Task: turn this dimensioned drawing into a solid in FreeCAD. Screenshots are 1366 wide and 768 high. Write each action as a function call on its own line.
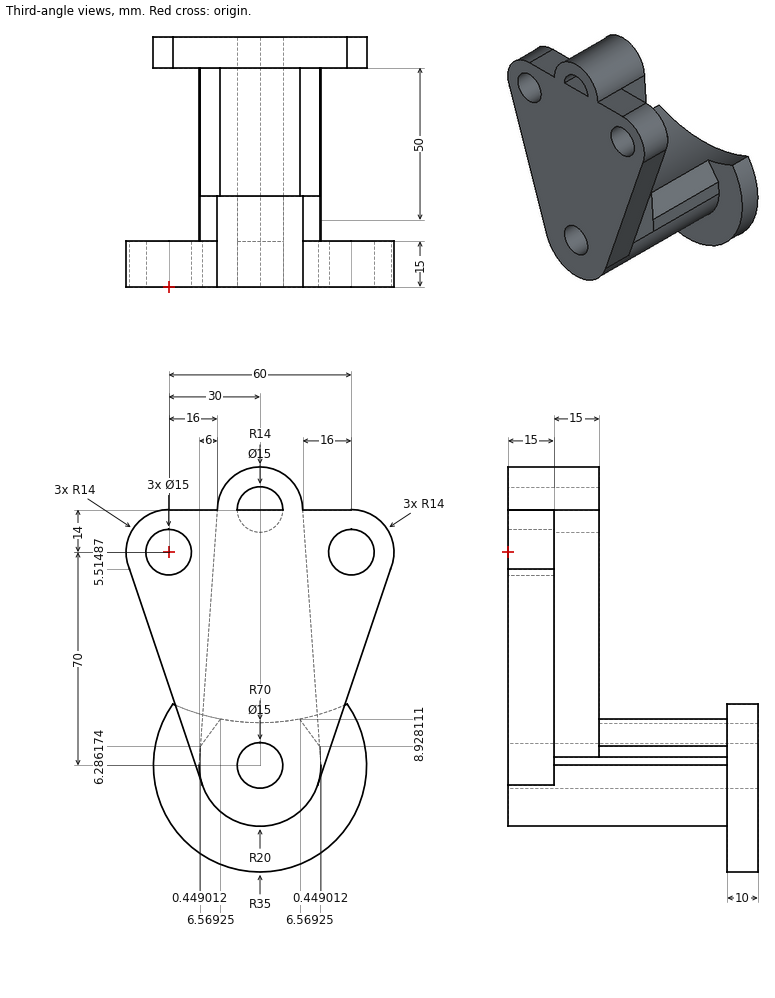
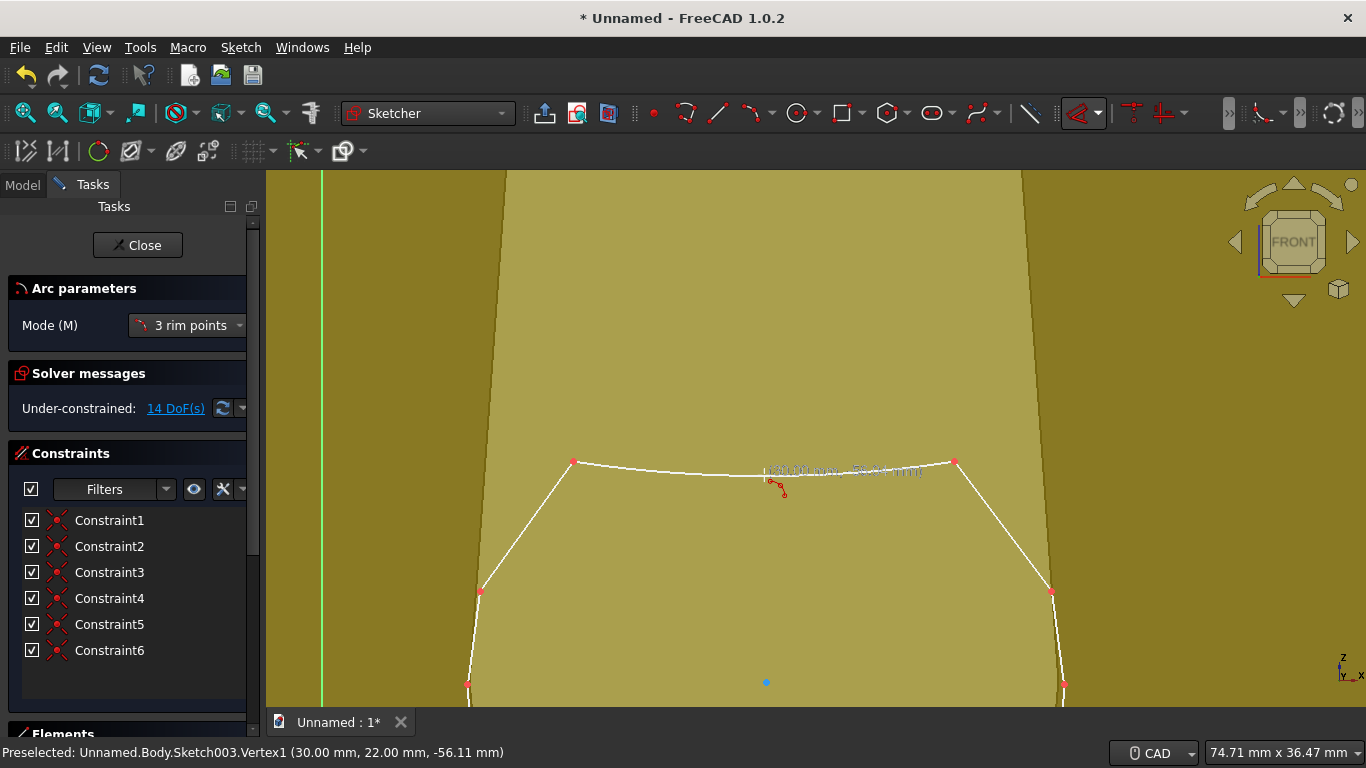
click(798, 114)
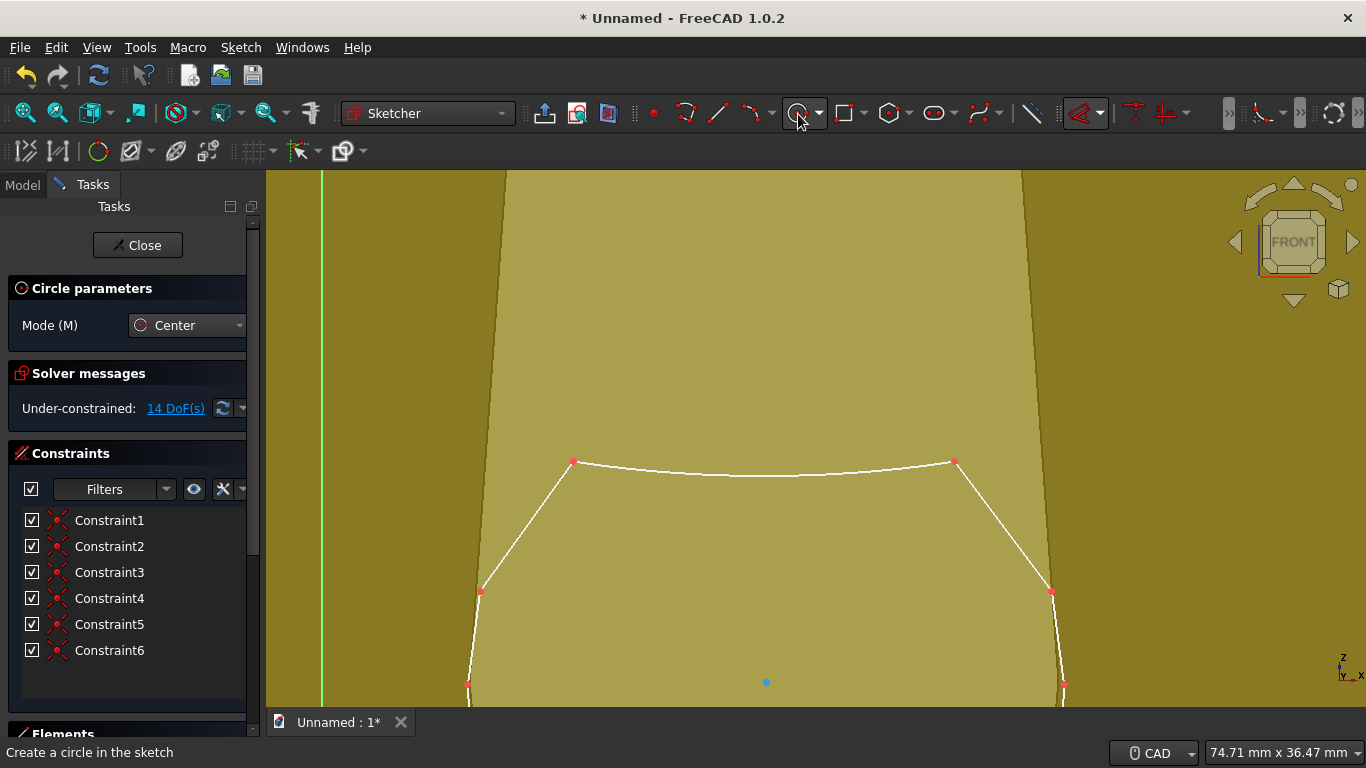
scroll(766, 479, down, 7)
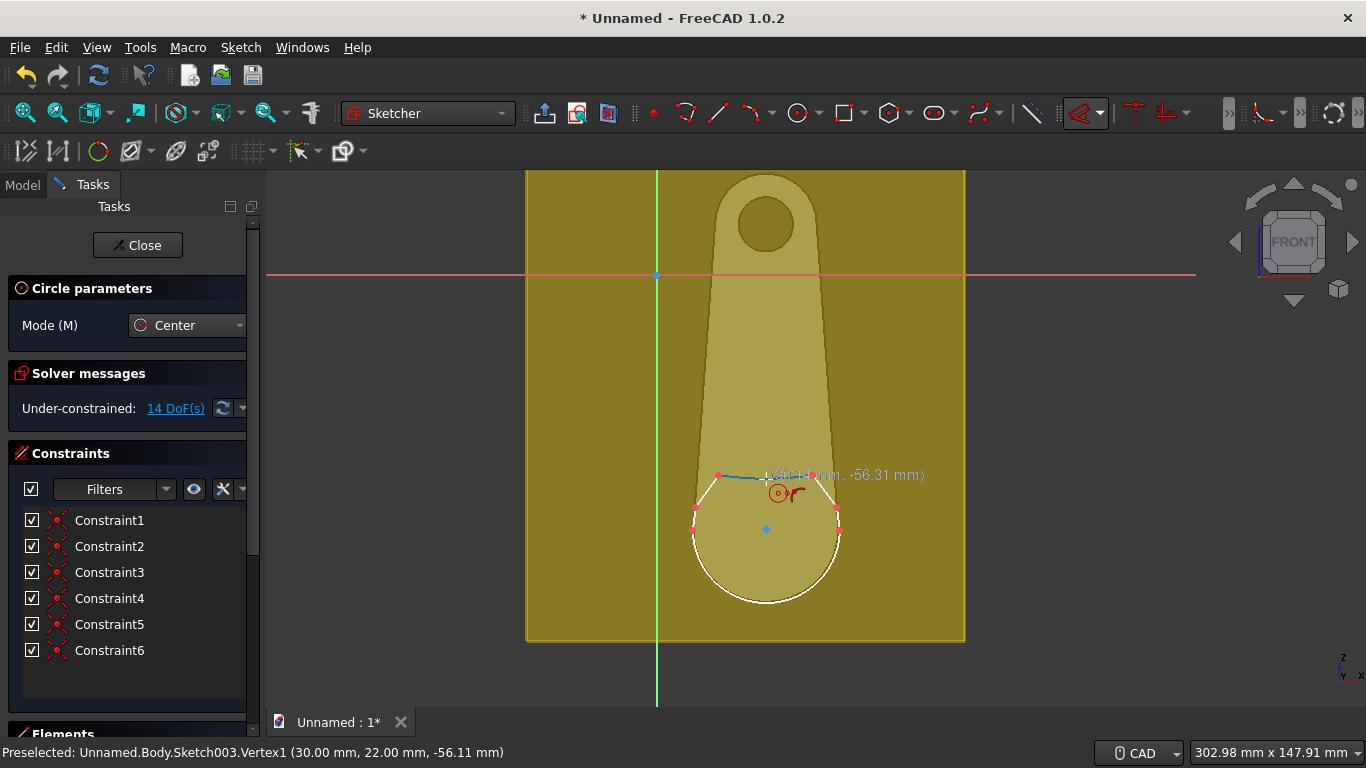
click(766, 529)
move(785, 510)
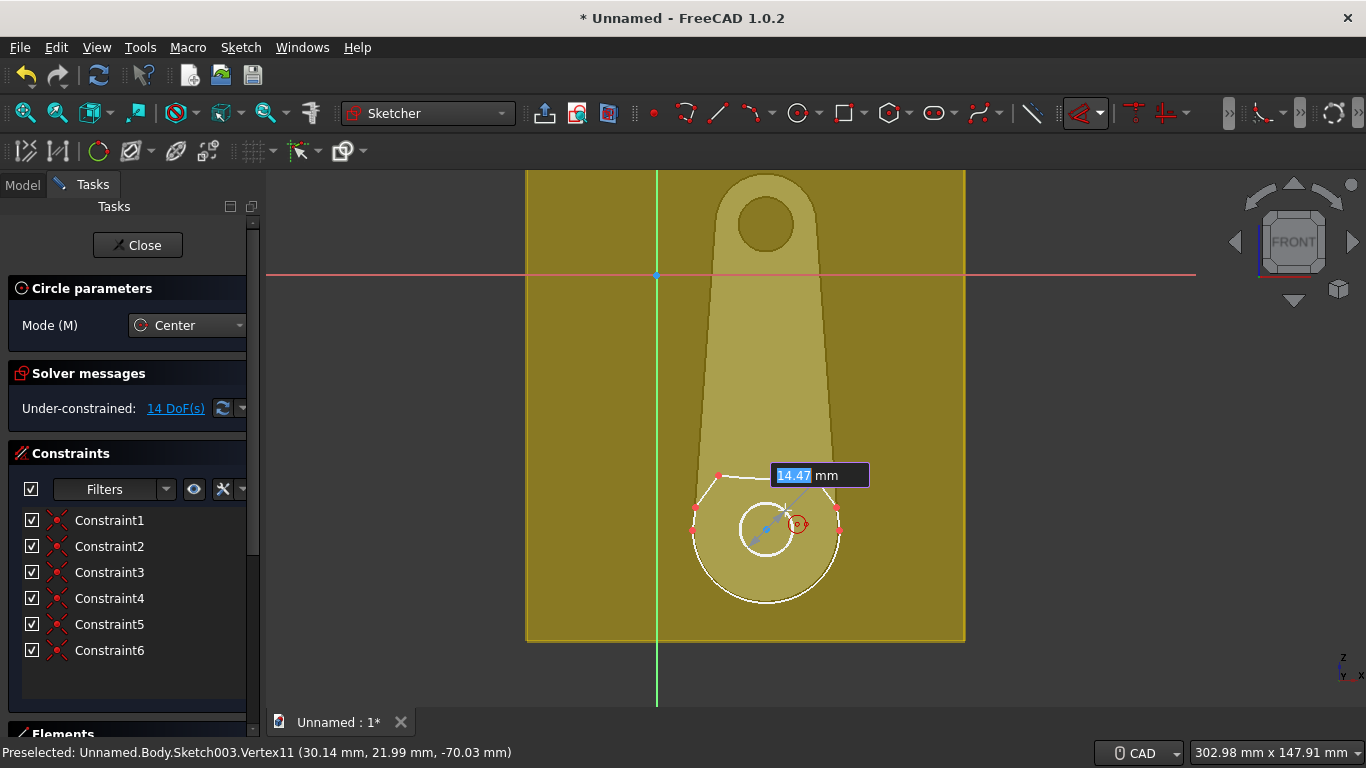
text(15)
key(Return)
key(Escape)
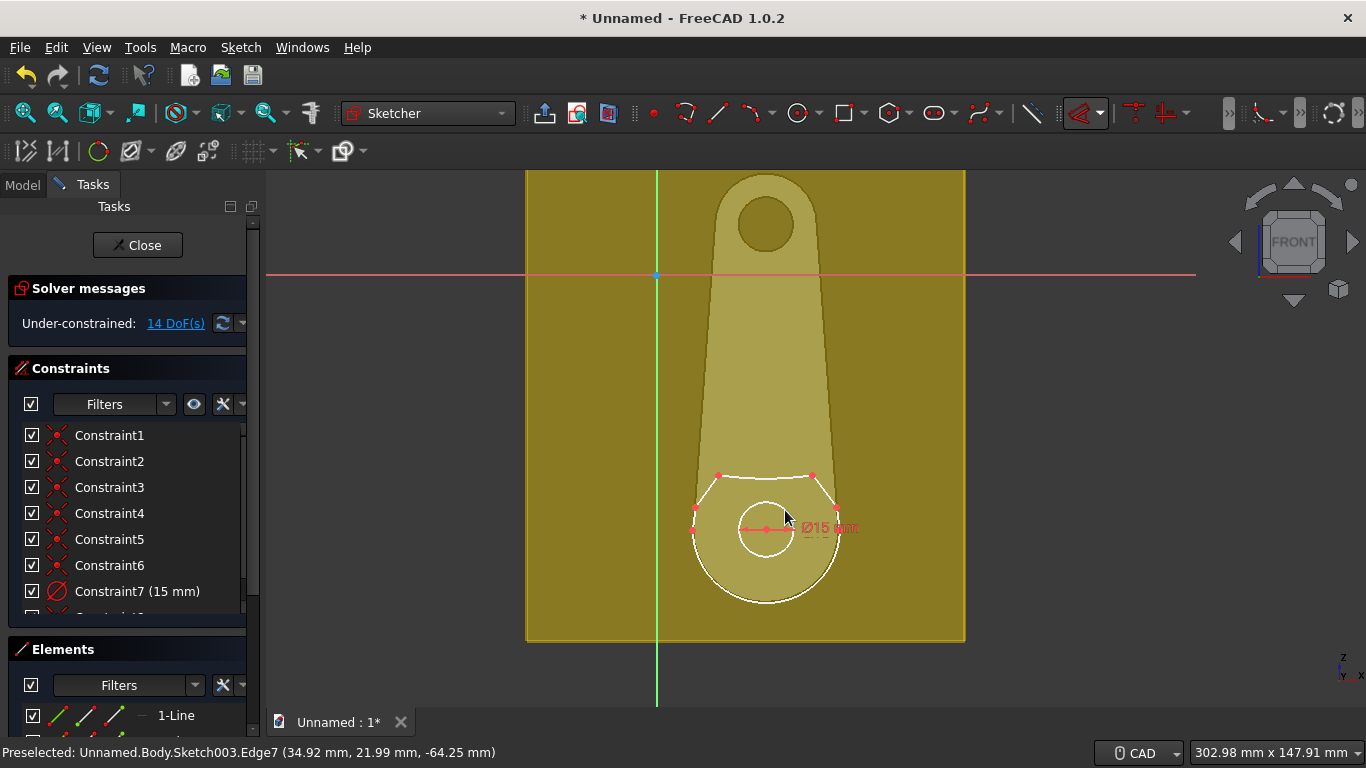
click(723, 589)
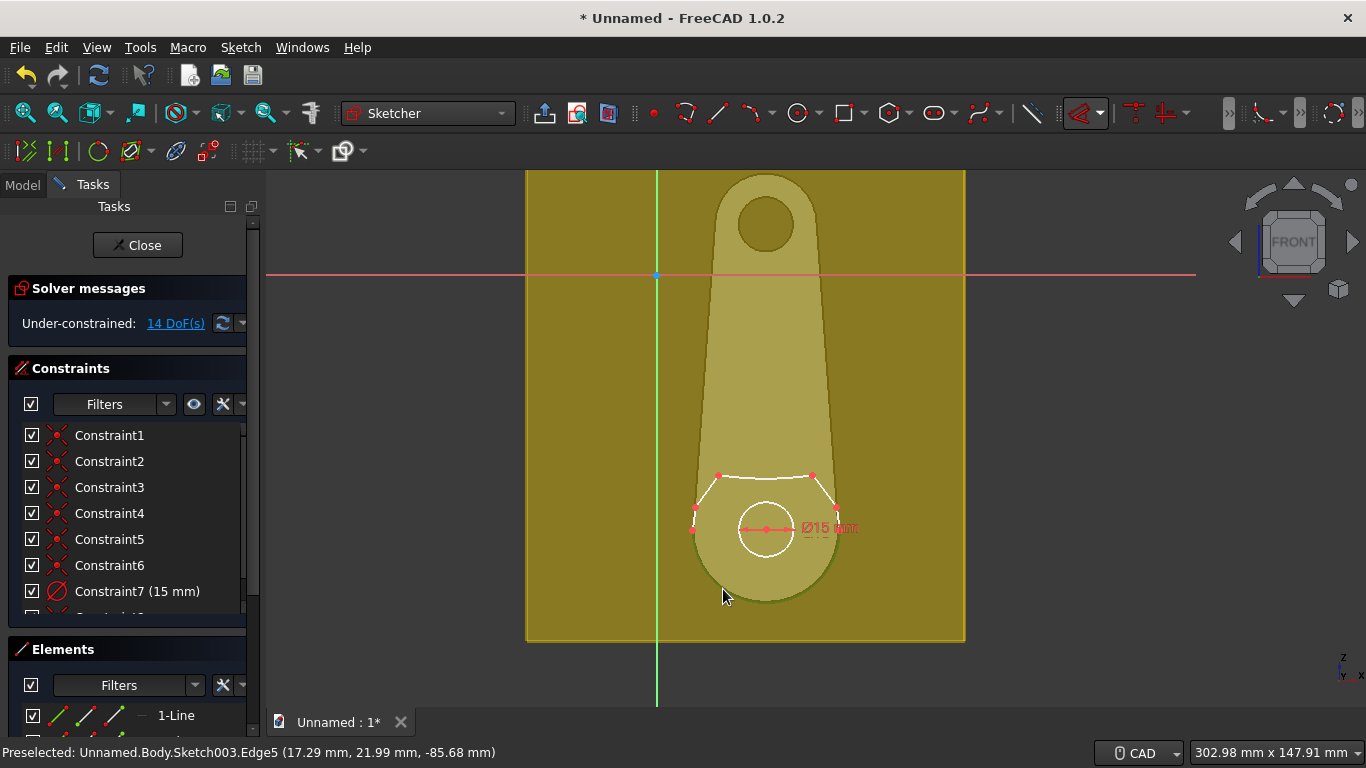
key(k)
key(r)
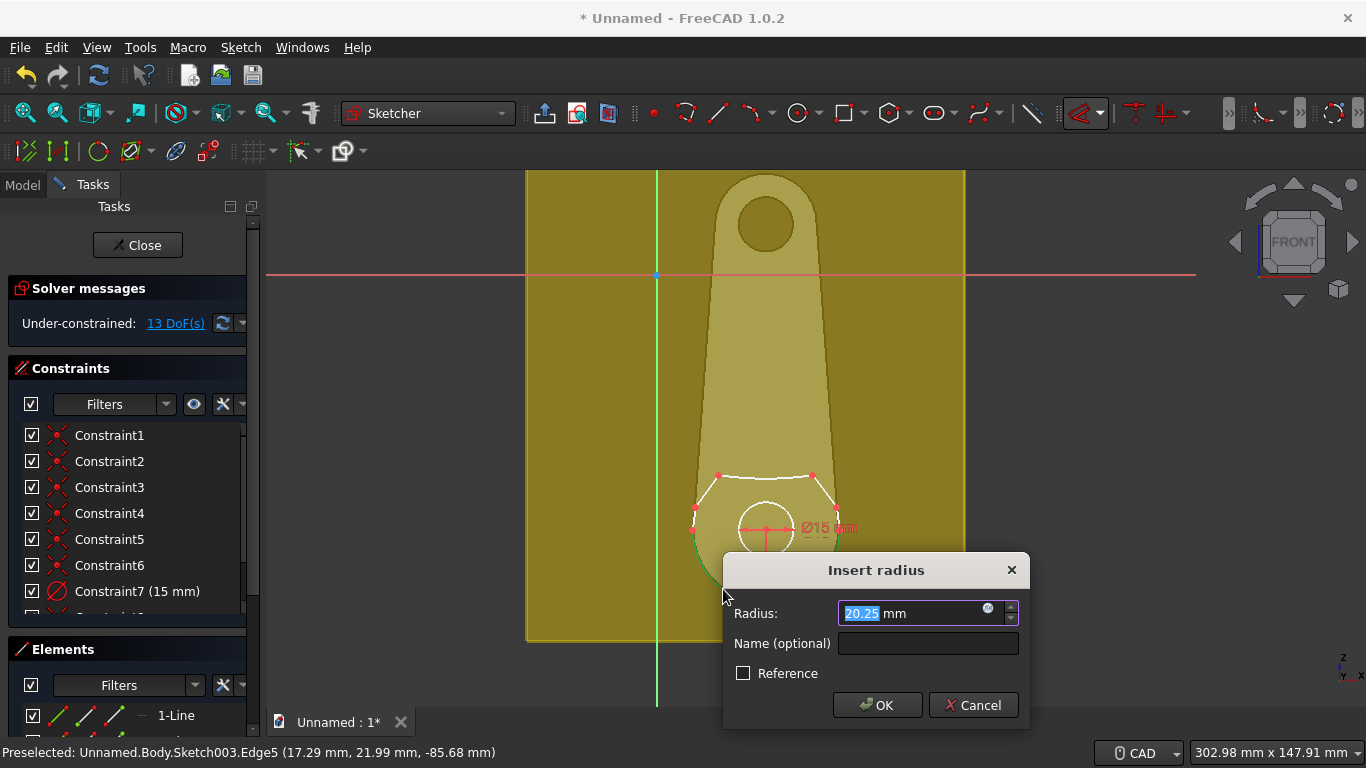
text(20)
key(Return)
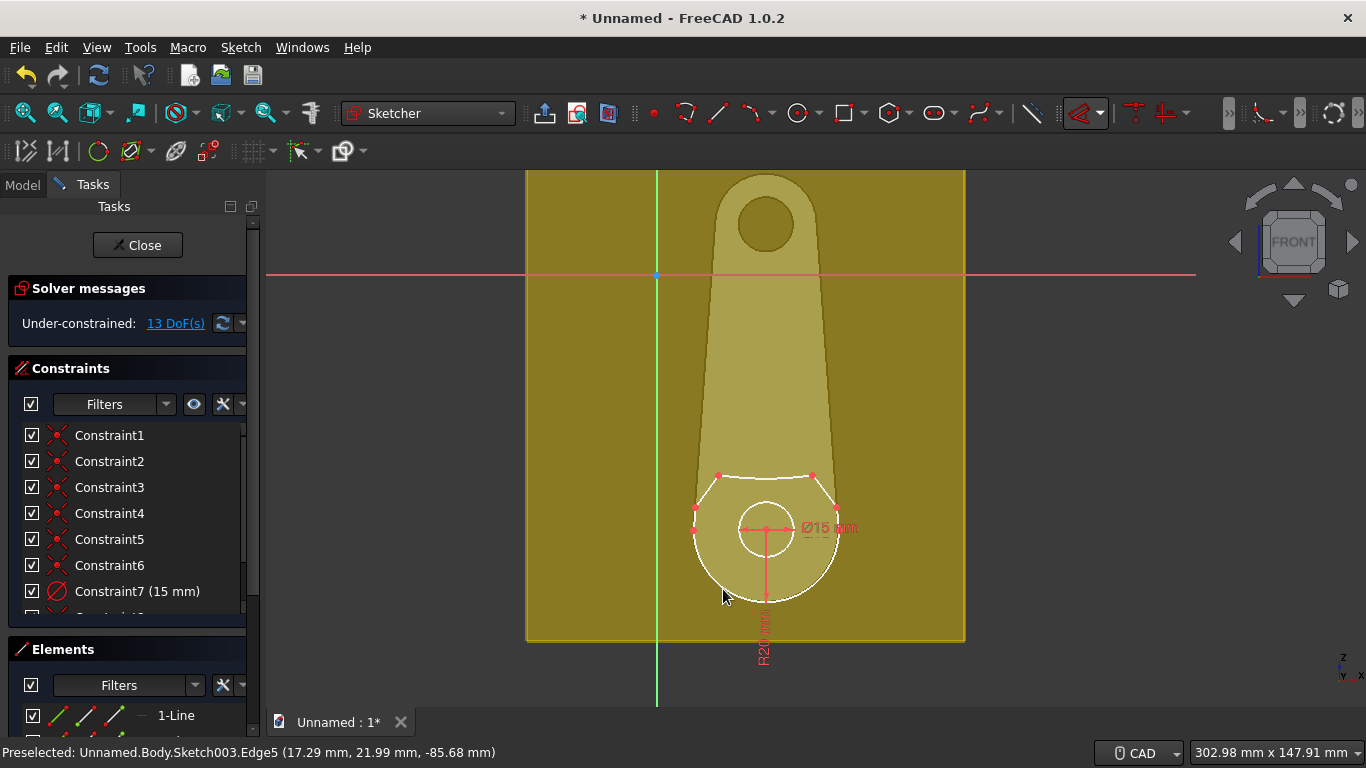
click(747, 478)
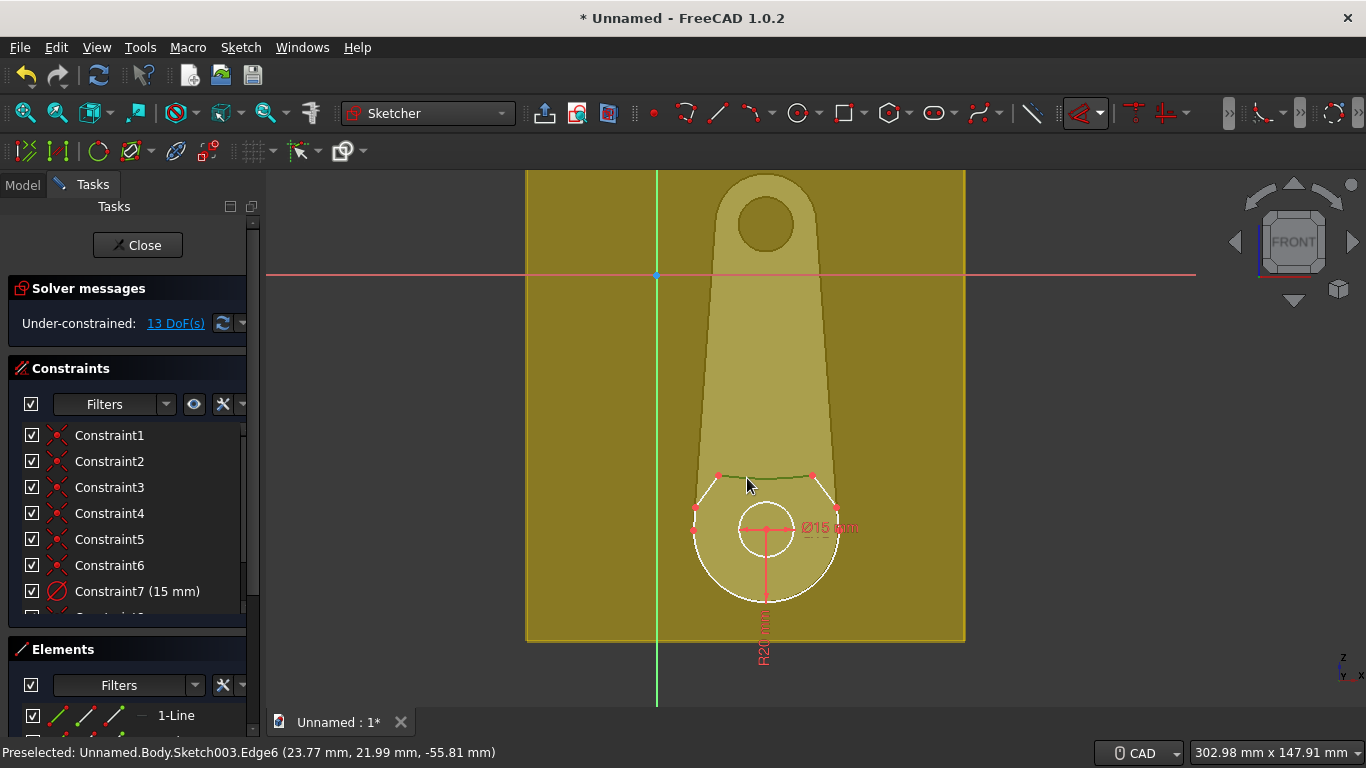
key(k)
key(r)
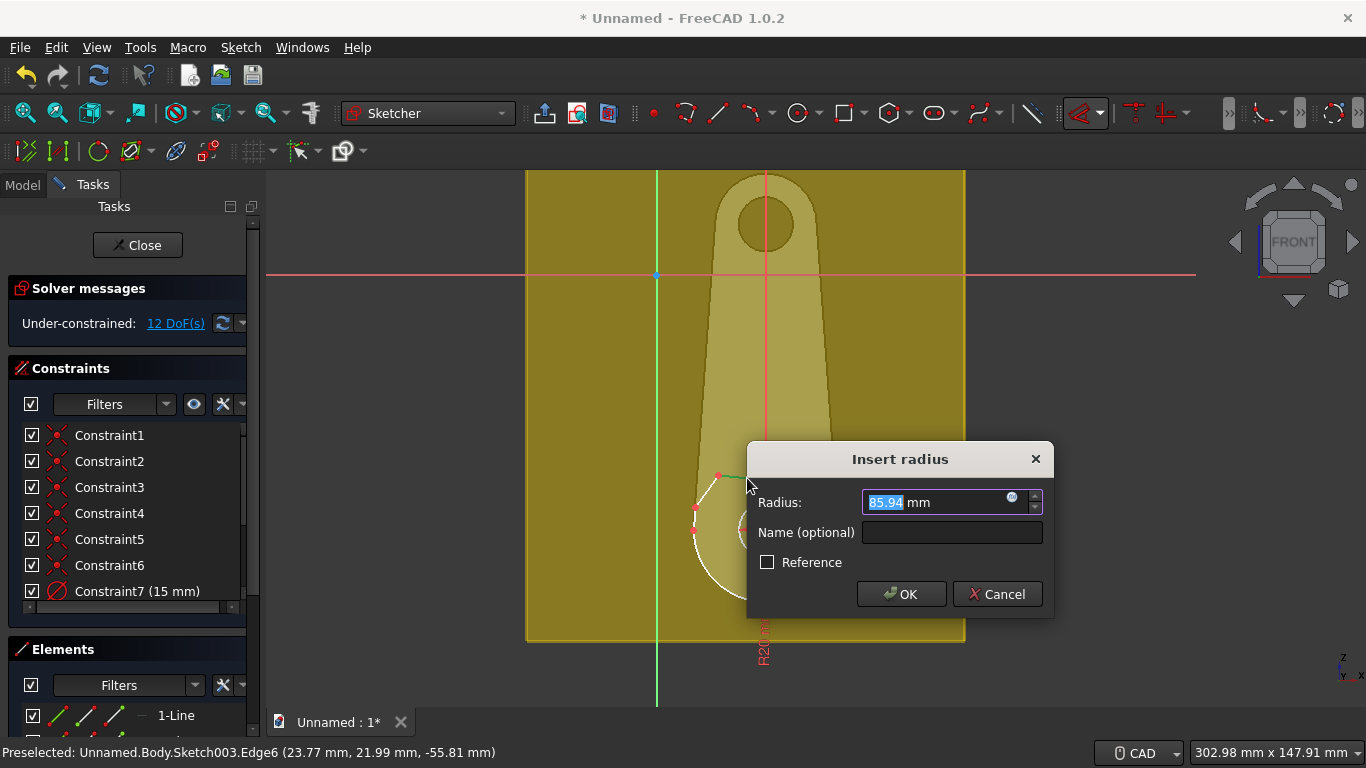
text(70)
key(Return)